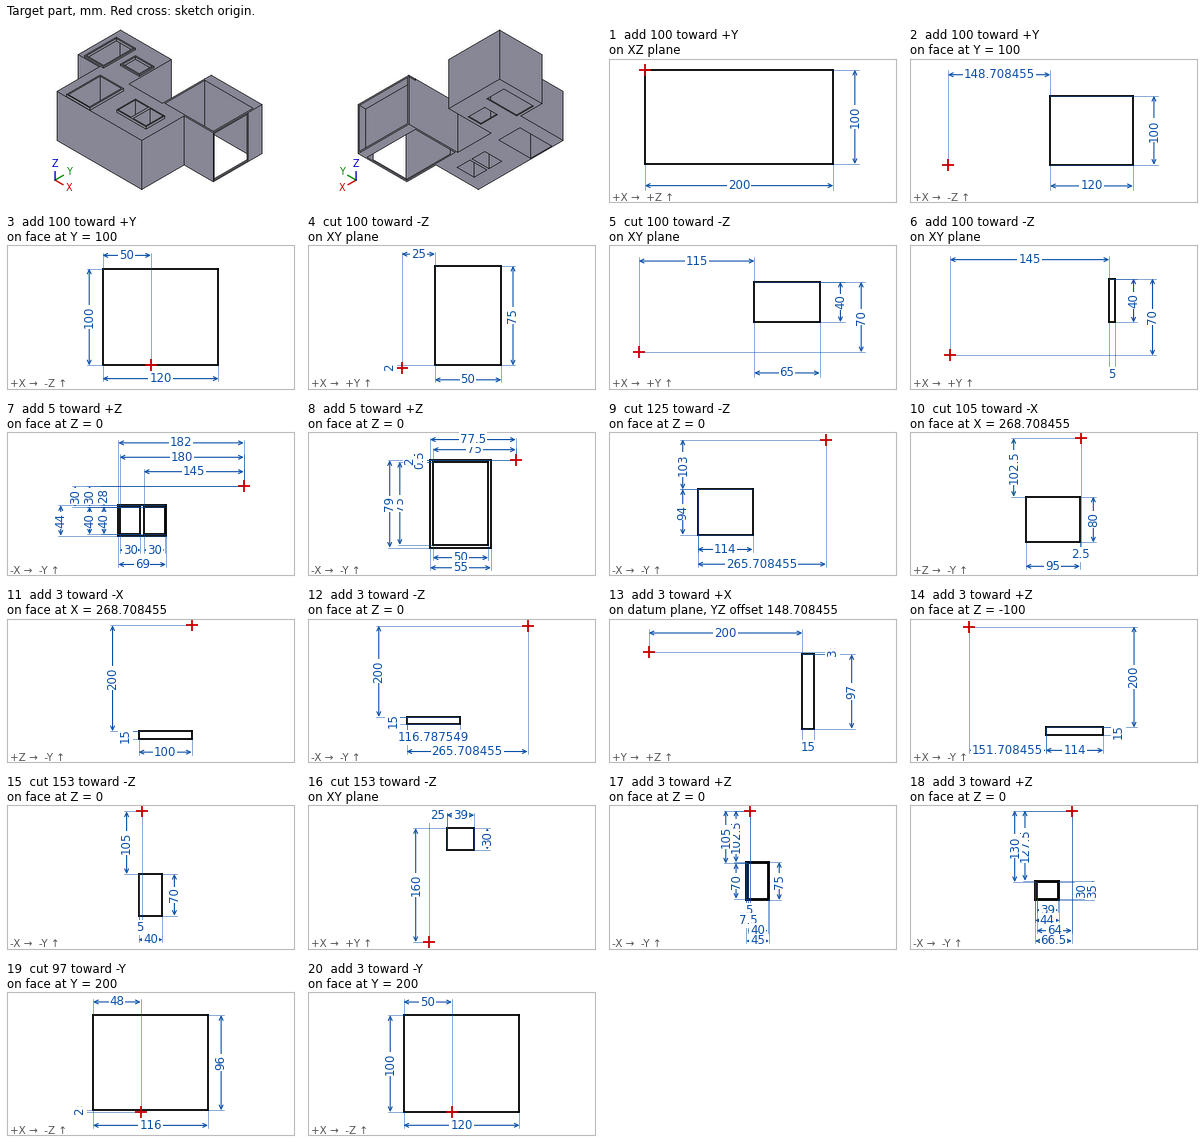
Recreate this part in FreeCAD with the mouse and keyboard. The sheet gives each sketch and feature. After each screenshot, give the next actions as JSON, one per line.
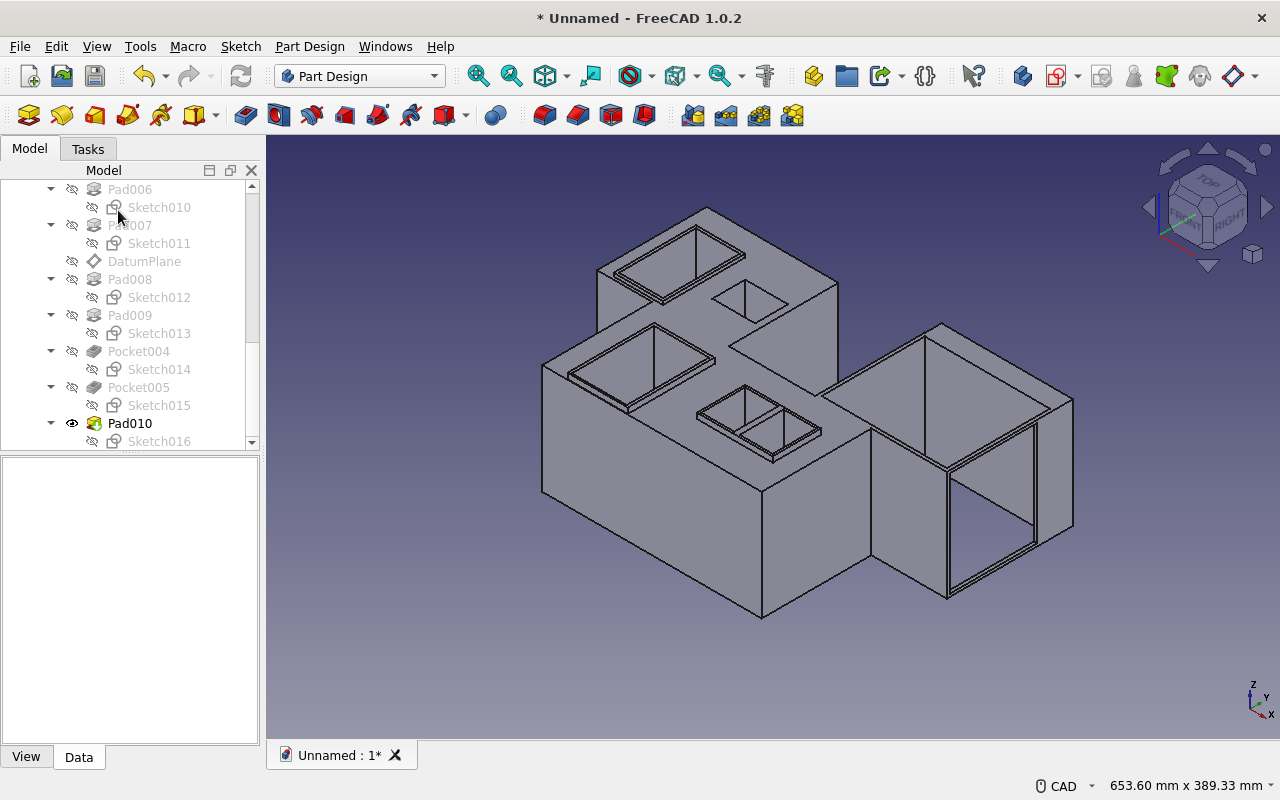
{"action": "left_click", "coordinate": [679, 424]}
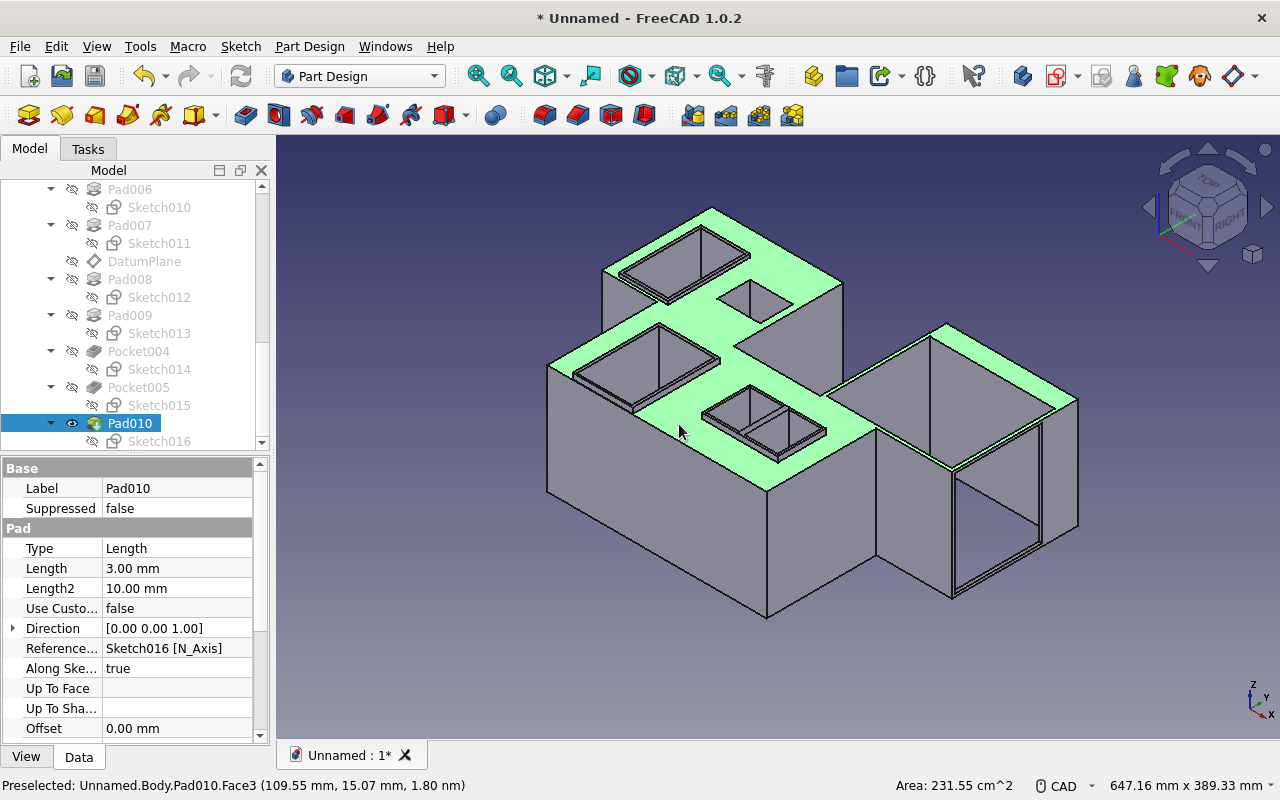
{"action": "left_click", "coordinate": [1056, 76]}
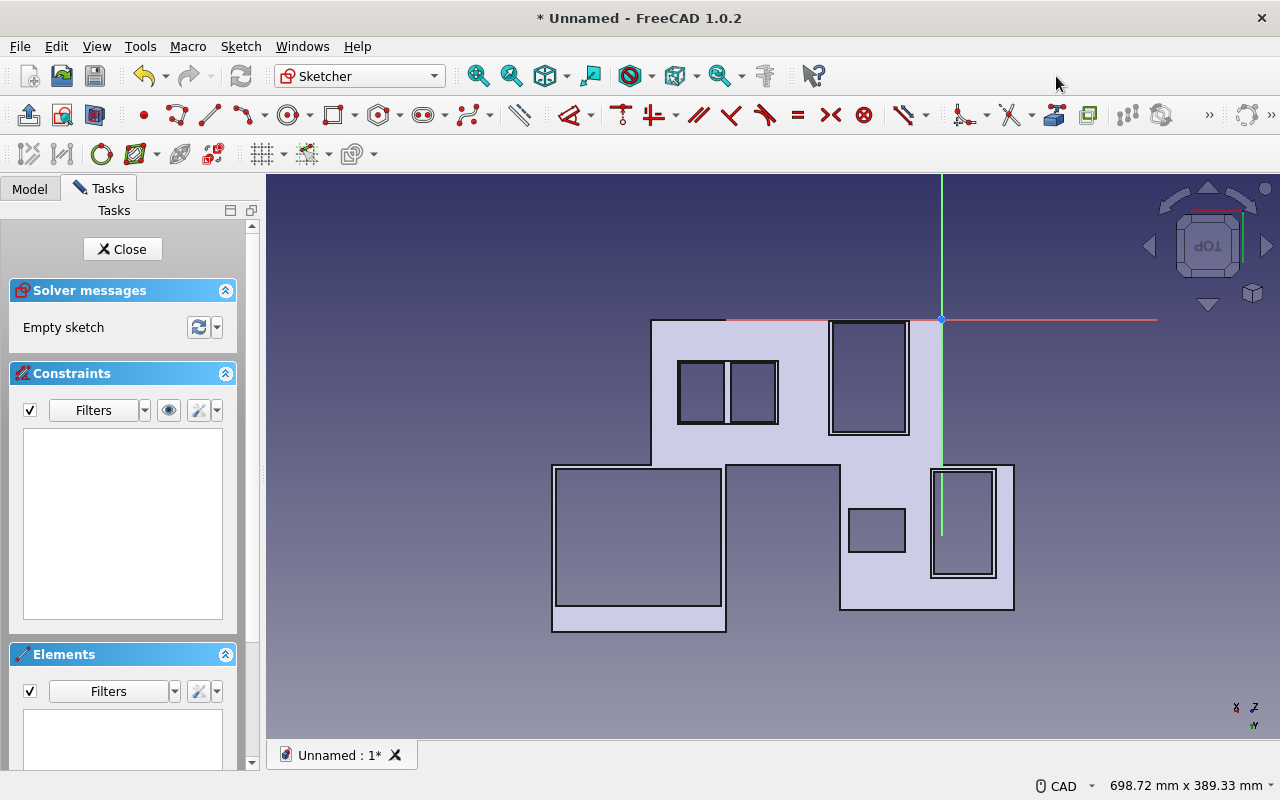
{"action": "left_click", "coordinate": [95, 116]}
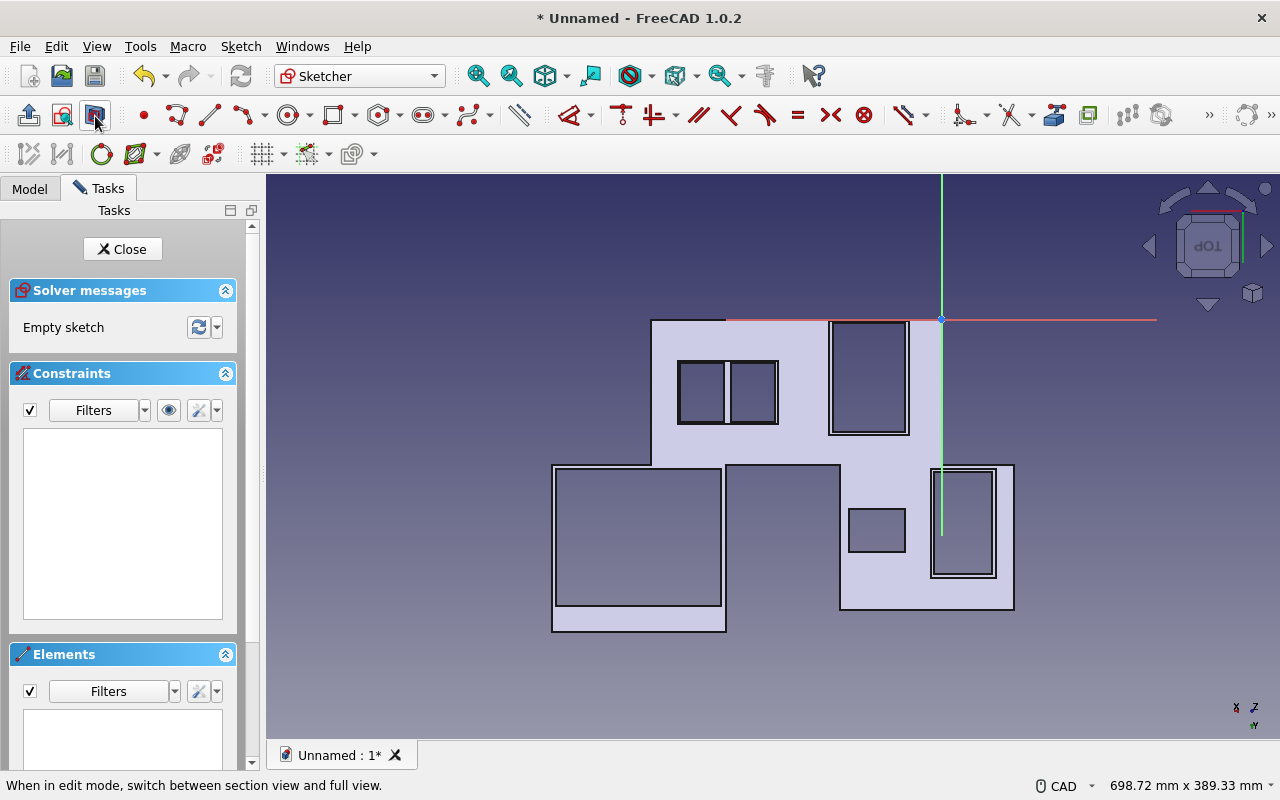
{"action": "scroll", "coordinate": [904, 542], "scroll_direction": "up", "scroll_amount": 10}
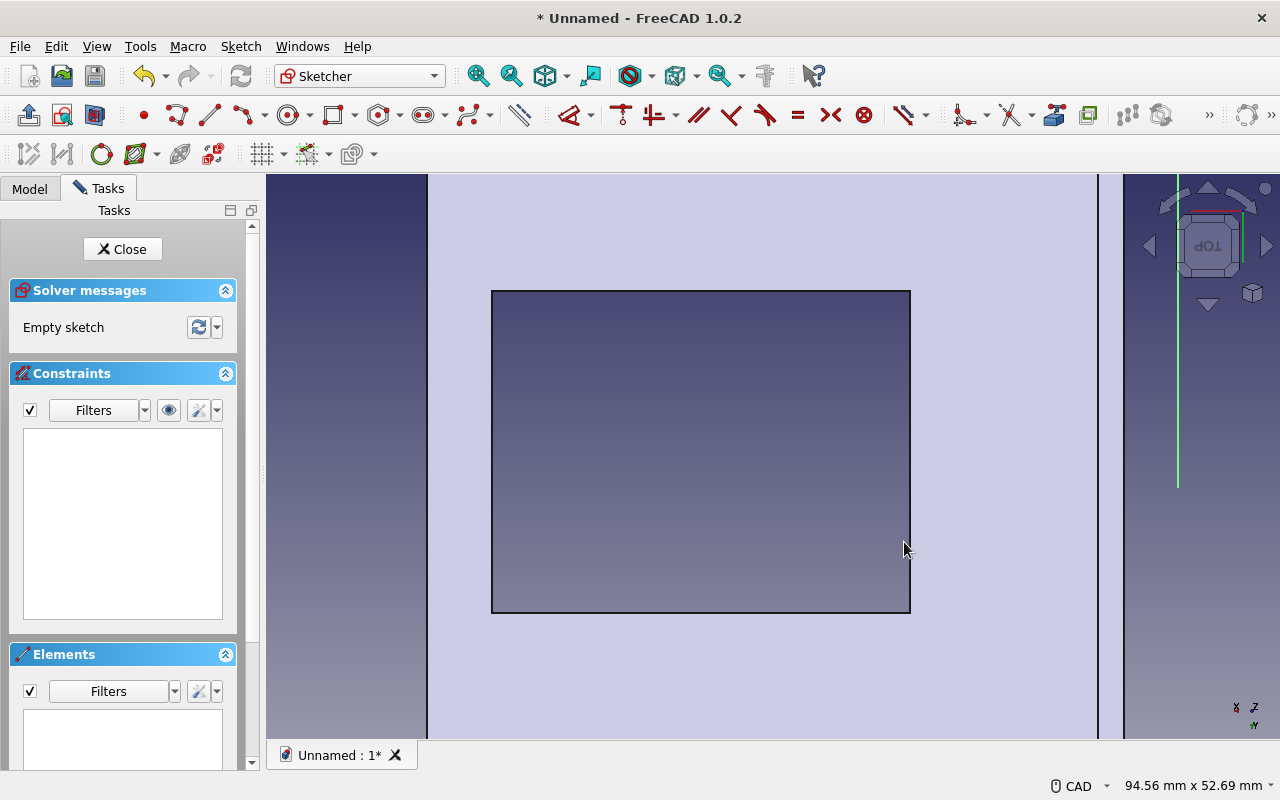
{"action": "left_click", "coordinate": [332, 116]}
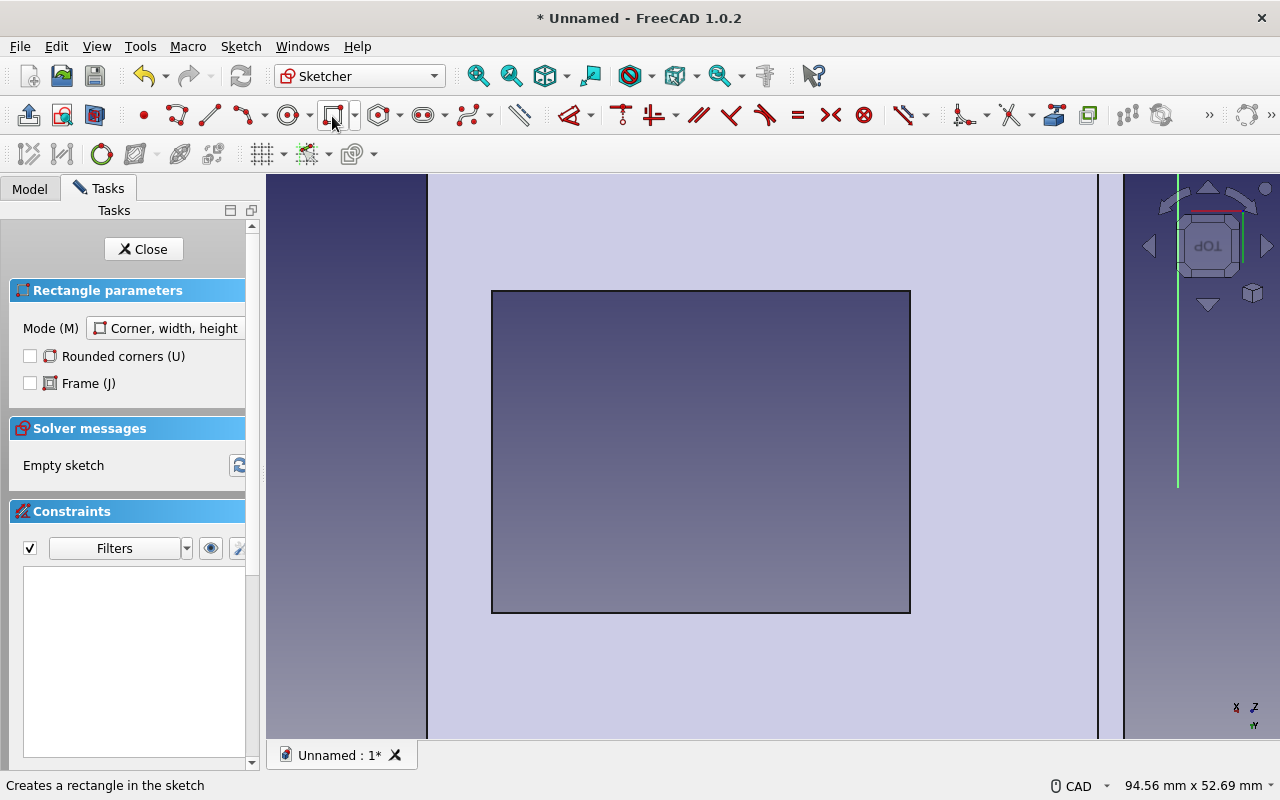
{"action": "left_click", "coordinate": [465, 264]}
{"action": "mouse_move", "coordinate": [937, 639]}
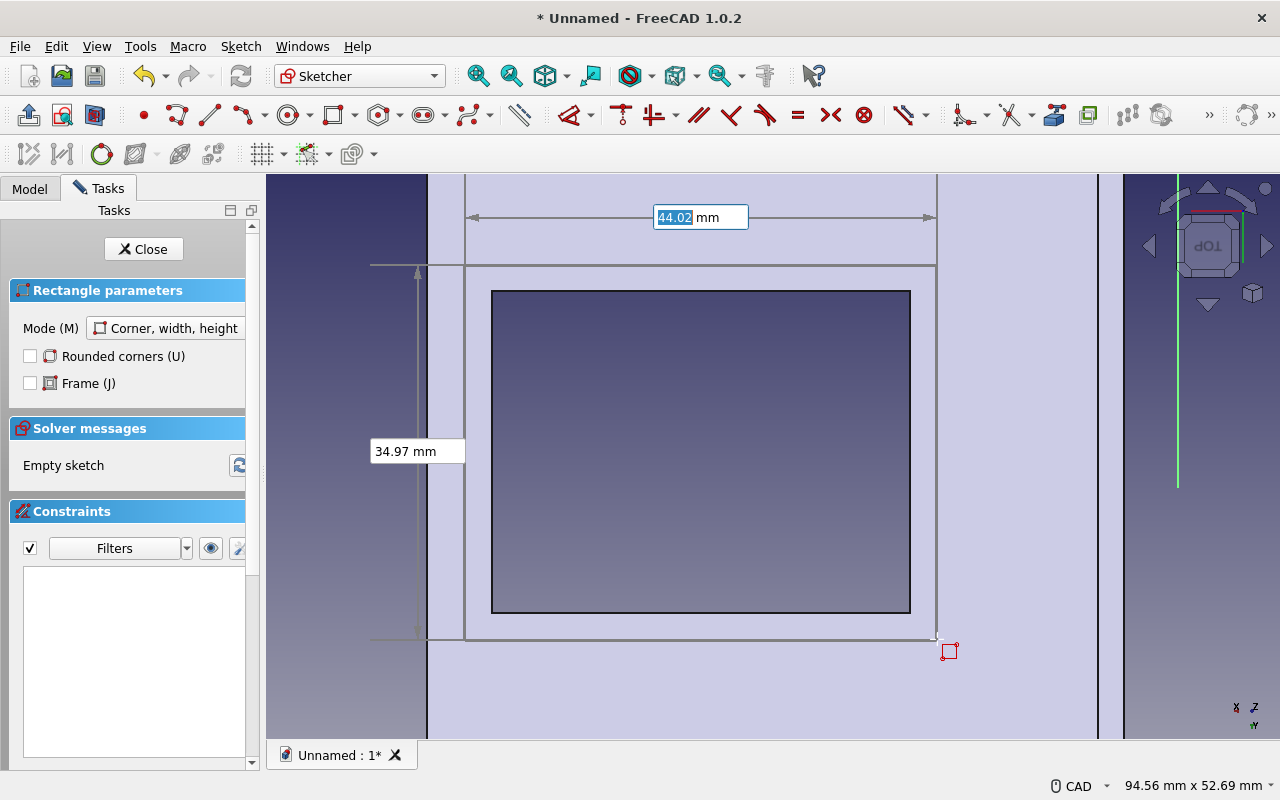
{"action": "type", "text": "44"}
{"action": "key", "text": "Tab"}
{"action": "type", "text": "35"}
{"action": "key", "text": "Return"}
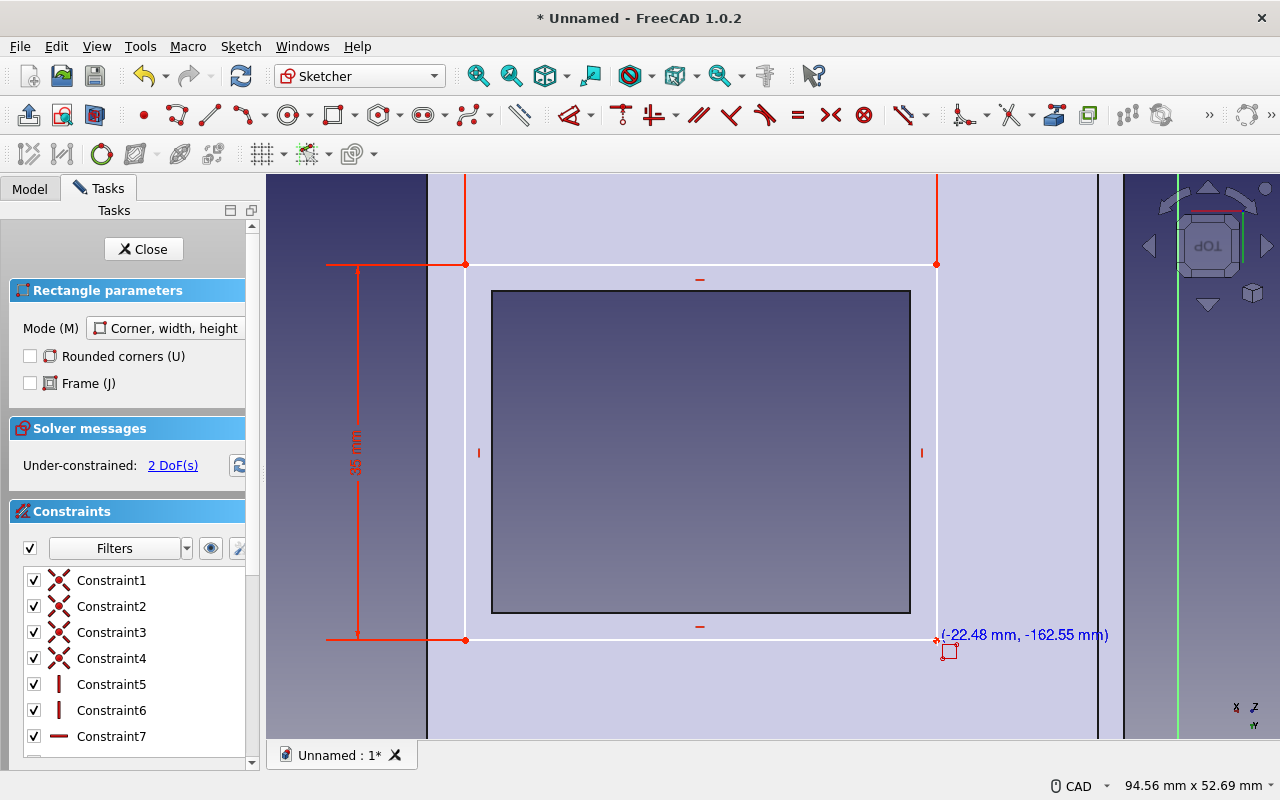
{"action": "left_click", "coordinate": [492, 291]}
{"action": "mouse_move", "coordinate": [910, 613]}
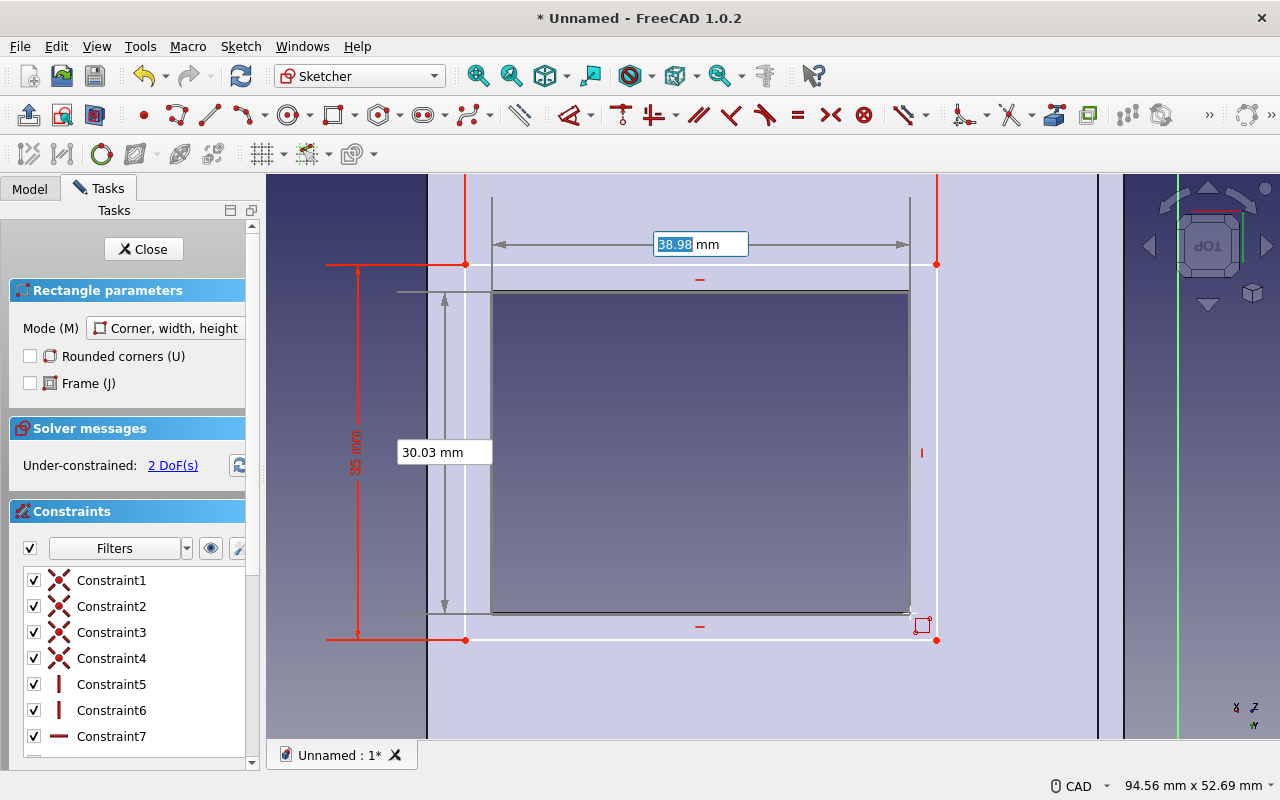
{"action": "type", "text": "39"}
{"action": "key", "text": "Tab"}
{"action": "type", "text": "30"}
{"action": "key", "text": "Return"}
{"action": "key", "text": "Escape"}